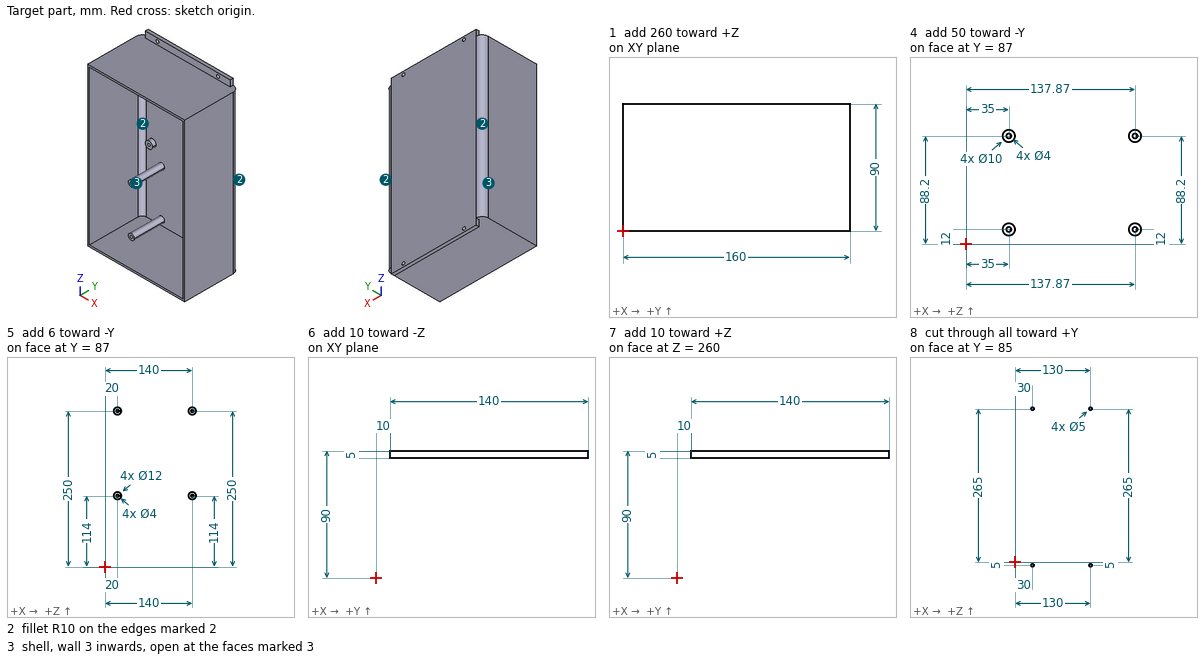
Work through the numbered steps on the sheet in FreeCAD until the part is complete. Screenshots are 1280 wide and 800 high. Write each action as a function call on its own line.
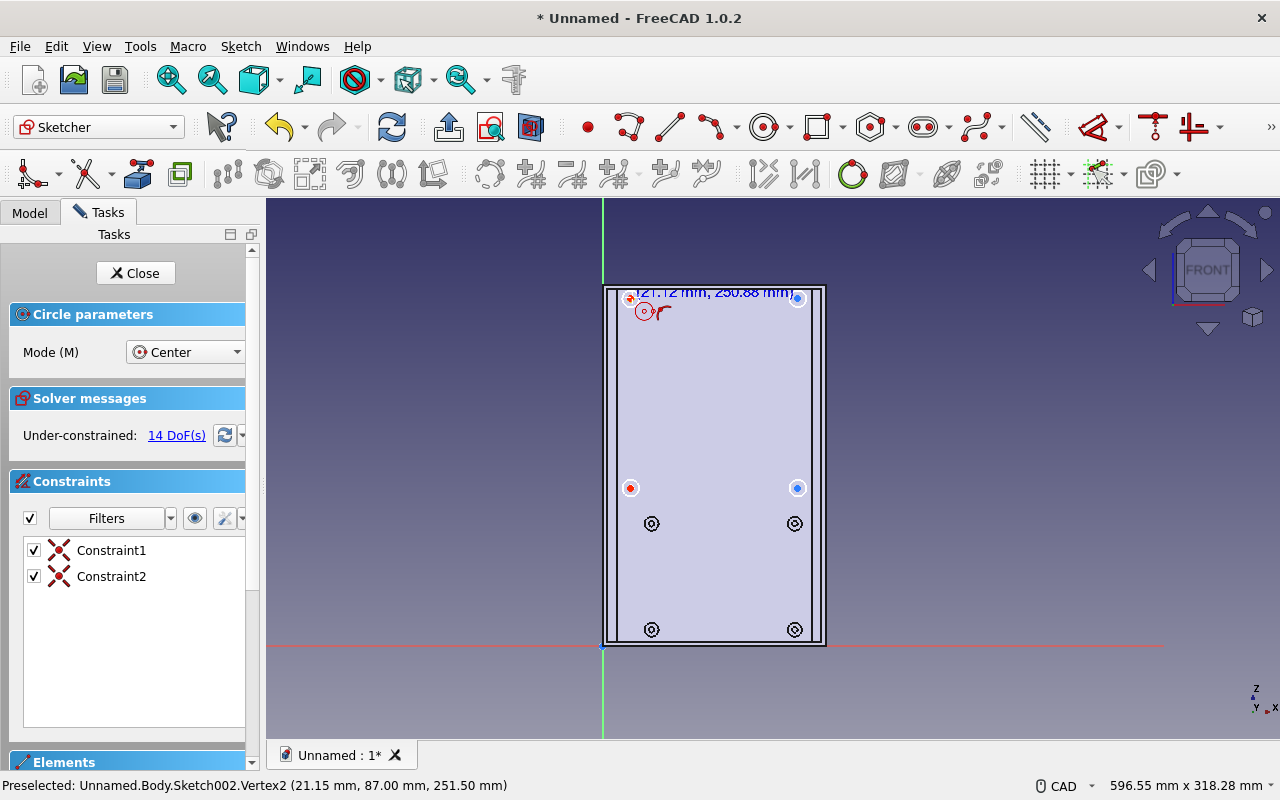
scroll(798, 488, up, 11)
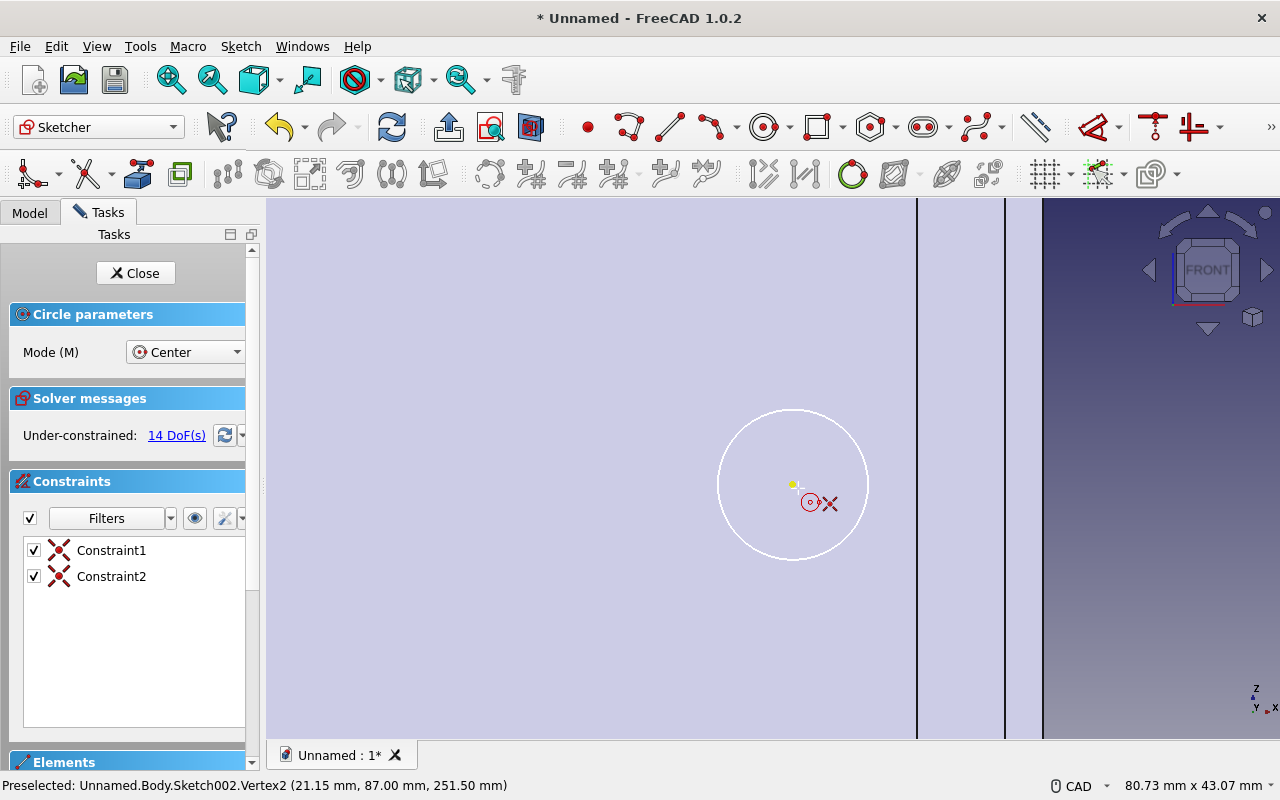
scroll(799, 489, down, 11)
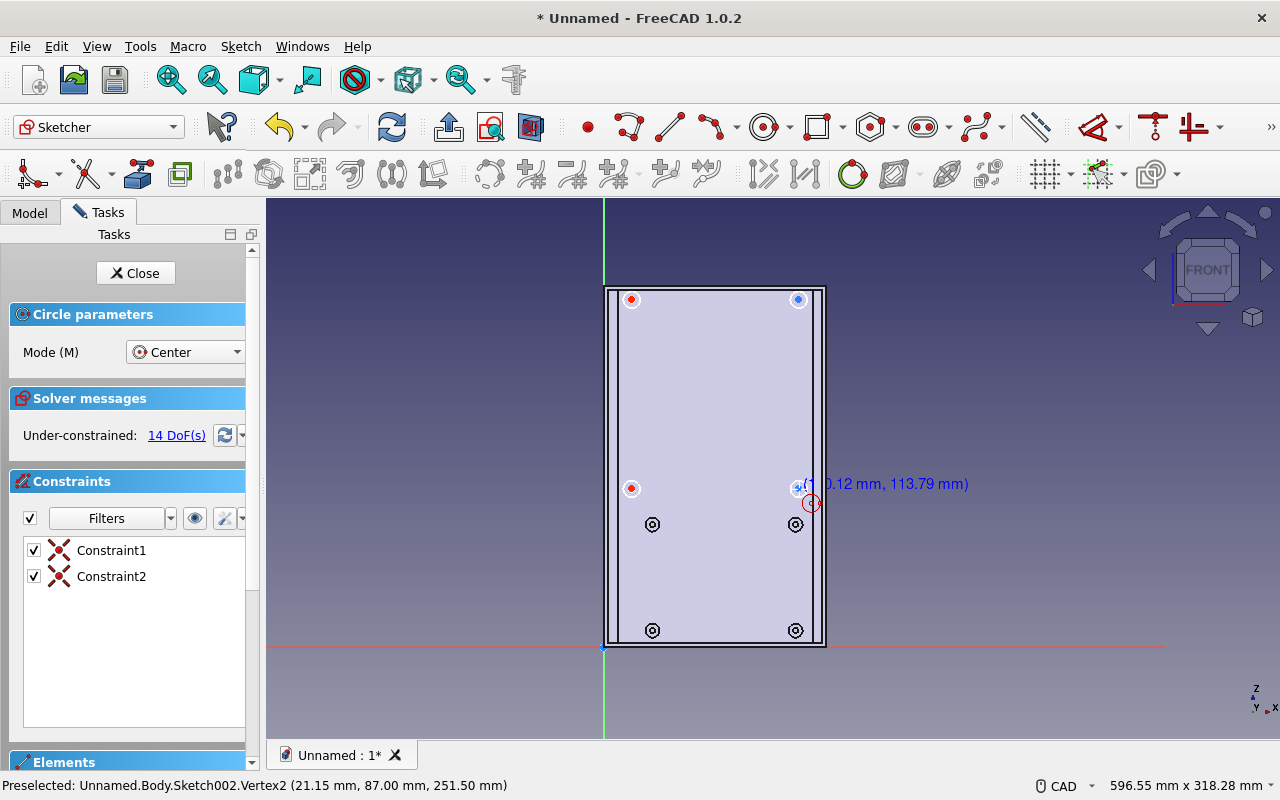
scroll(799, 489, up, 4)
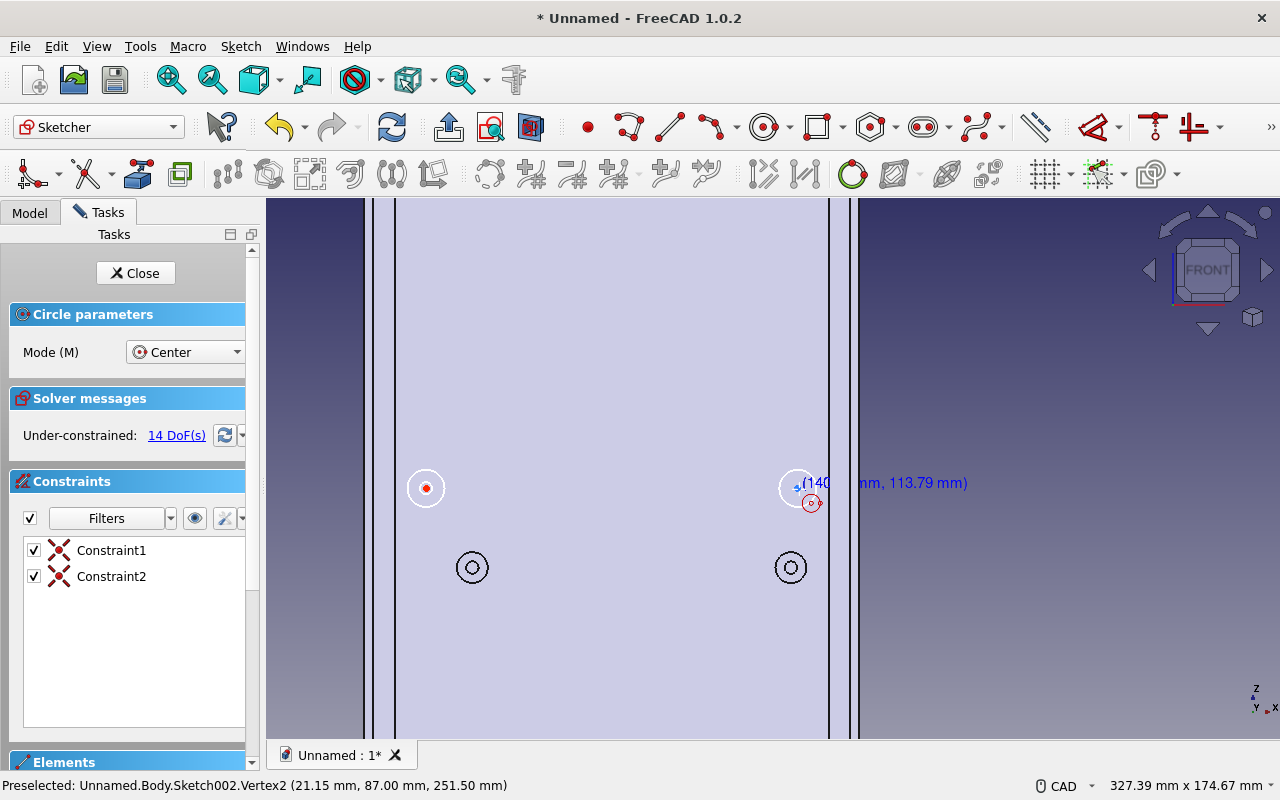
click(798, 488)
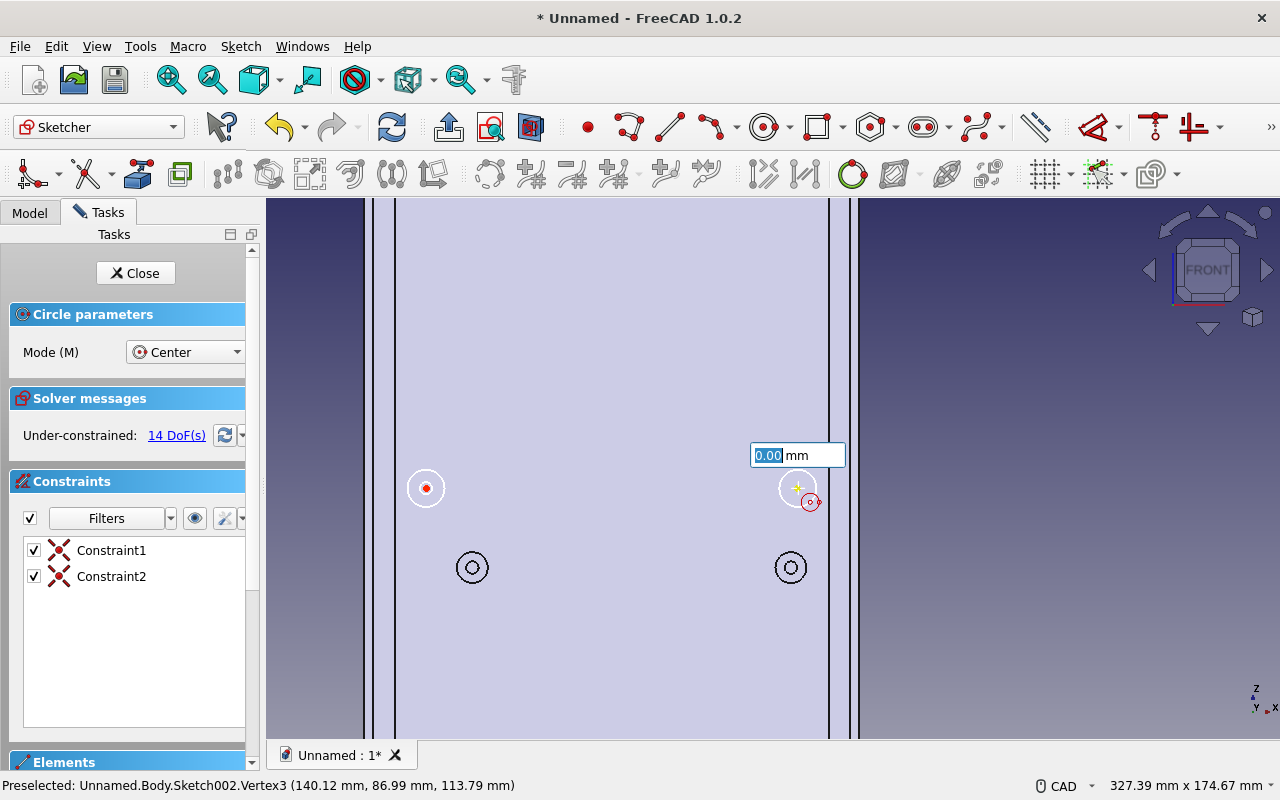
scroll(802, 483, up, 5)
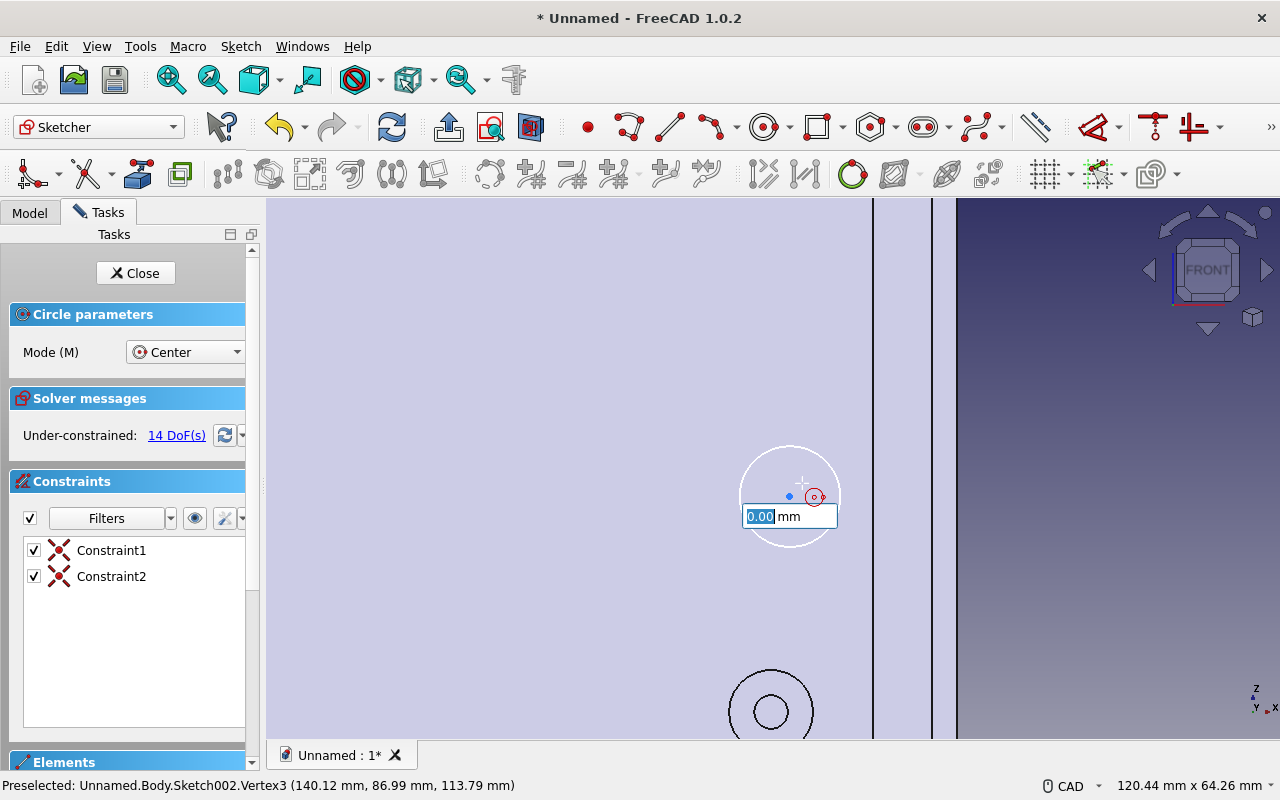
click(801, 483)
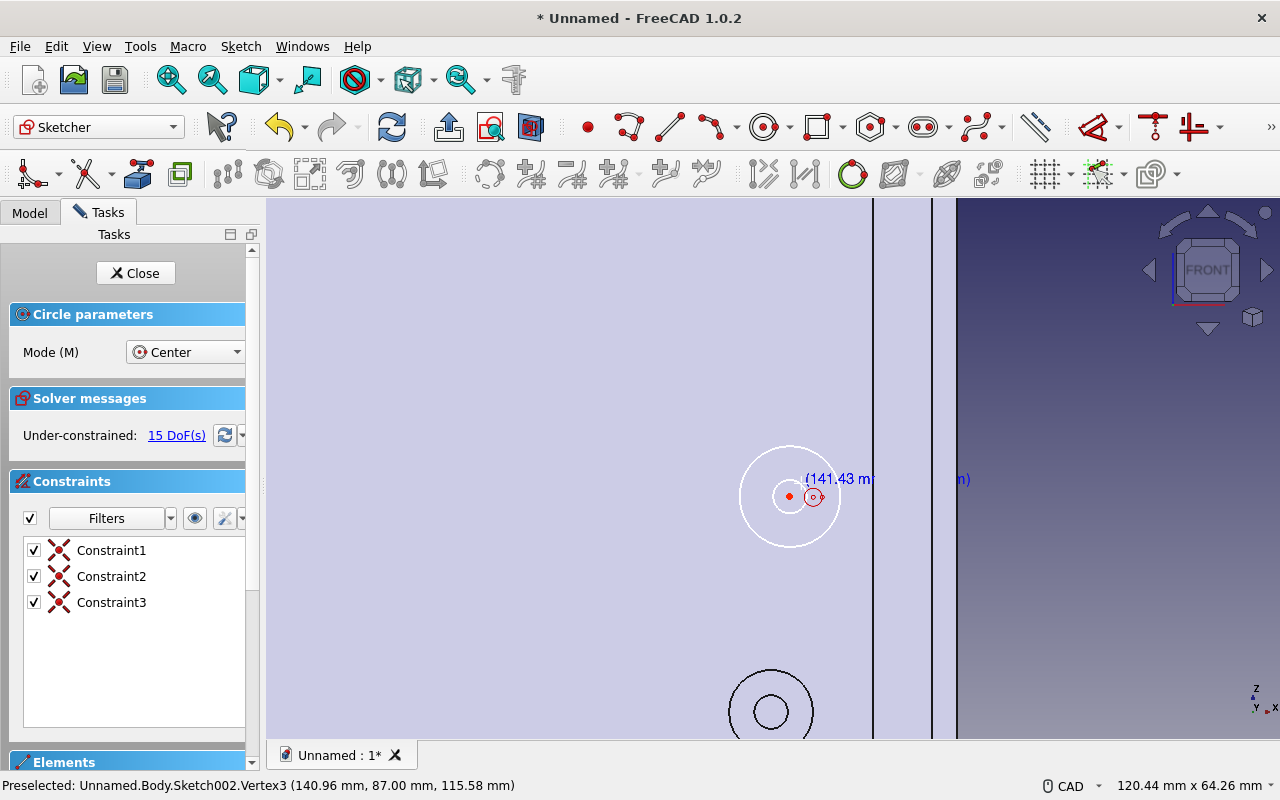
scroll(799, 487, down, 9)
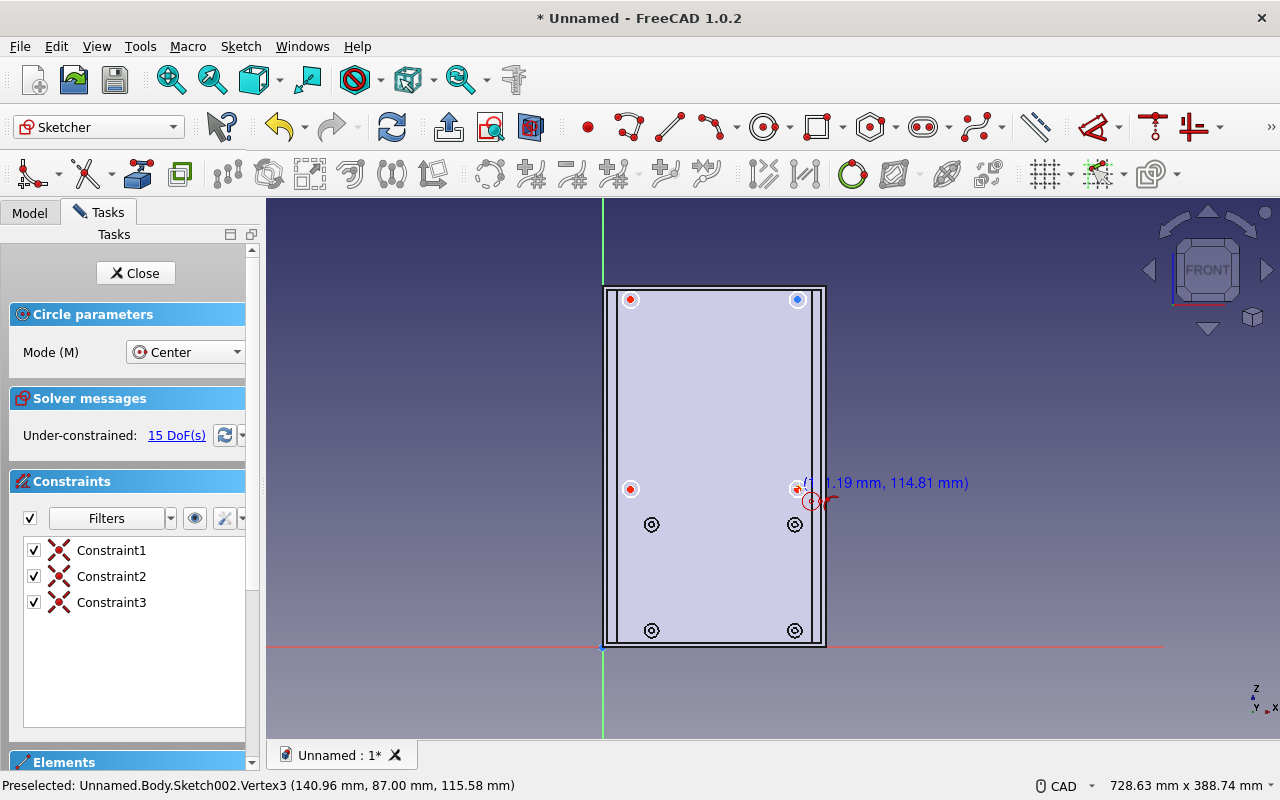
scroll(798, 299, up, 11)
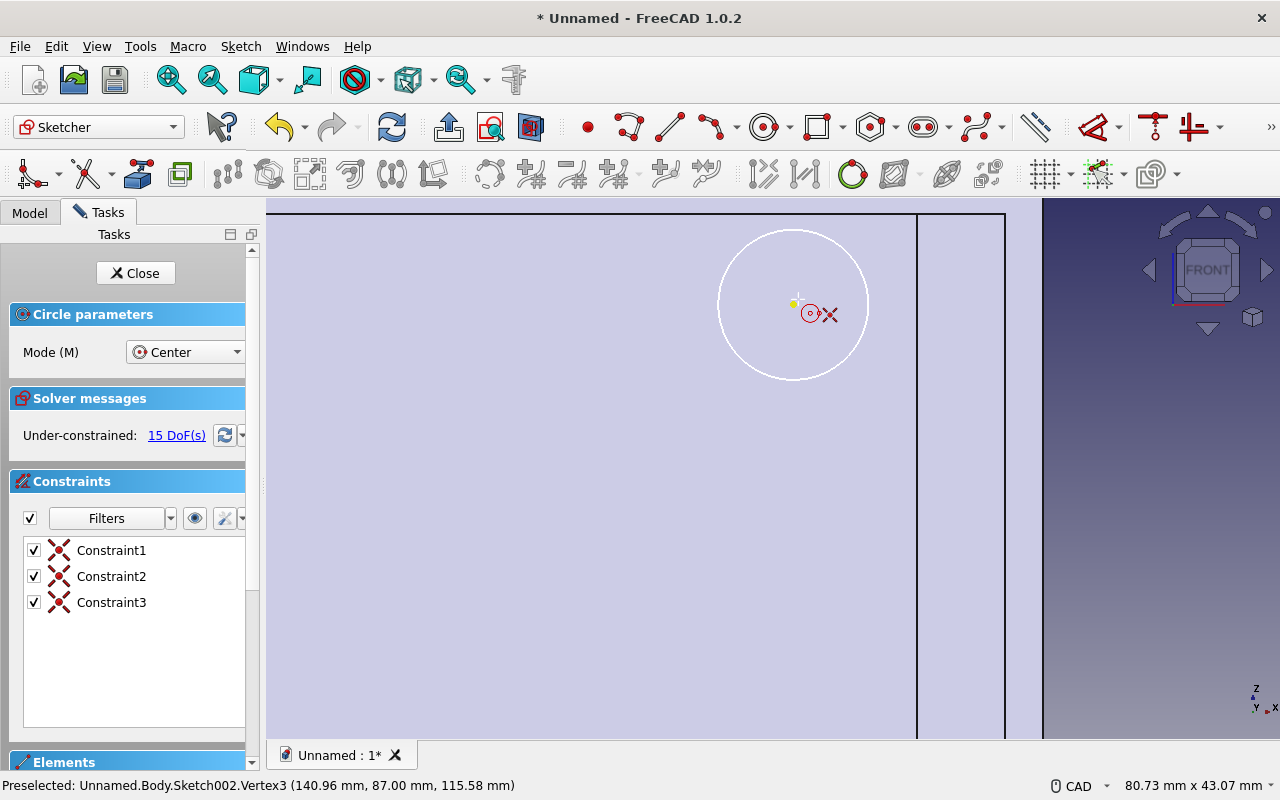
scroll(798, 298, down, 11)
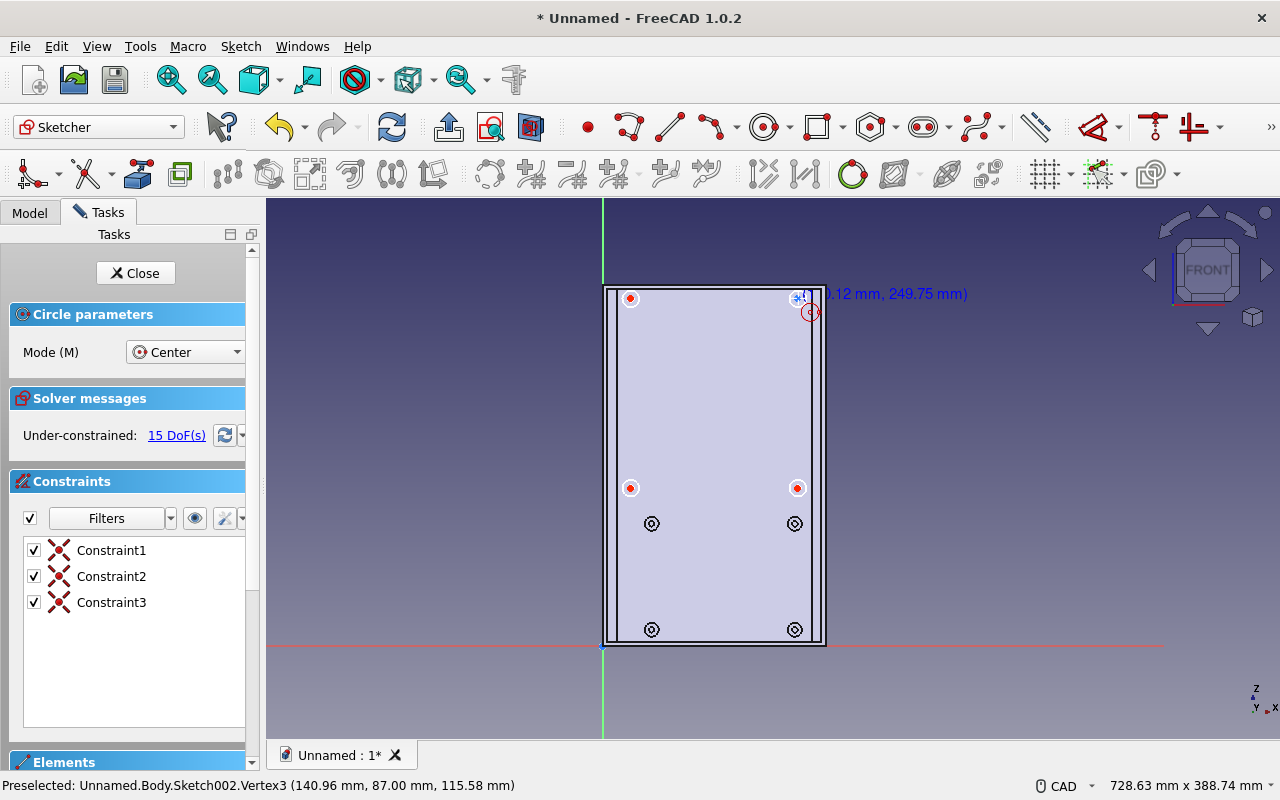
scroll(798, 299, up, 4)